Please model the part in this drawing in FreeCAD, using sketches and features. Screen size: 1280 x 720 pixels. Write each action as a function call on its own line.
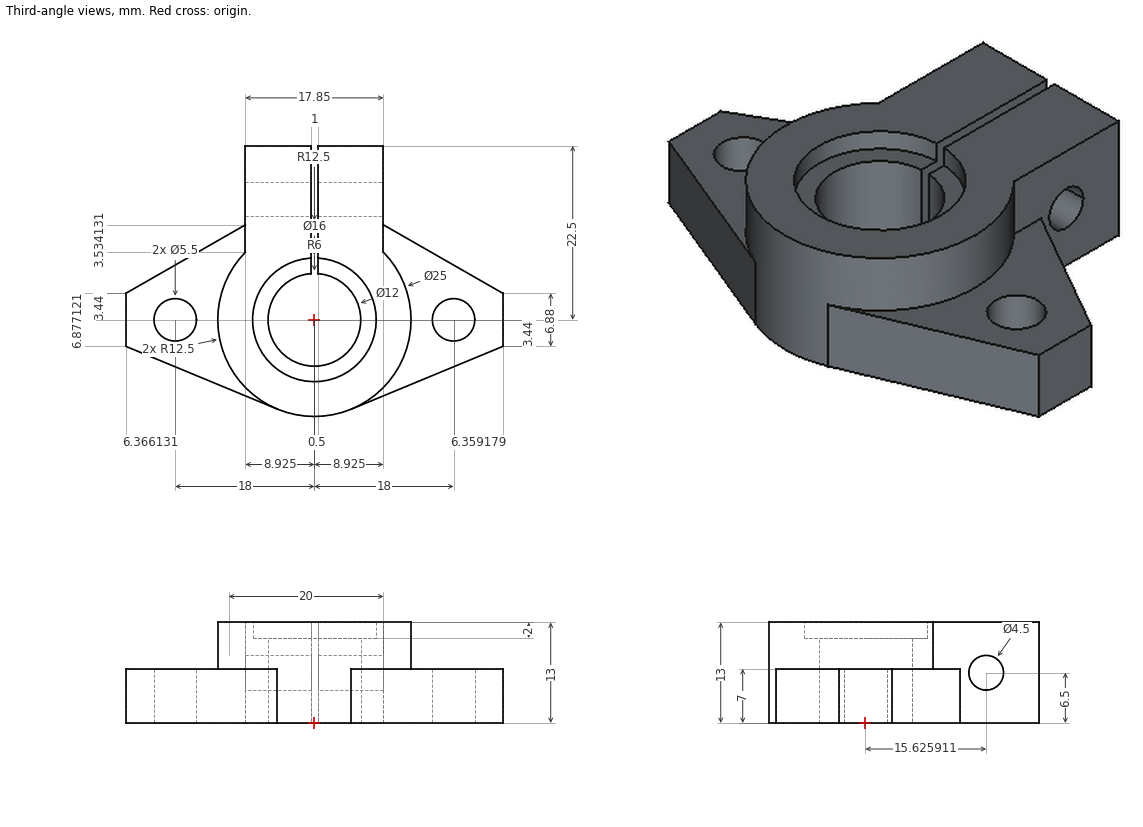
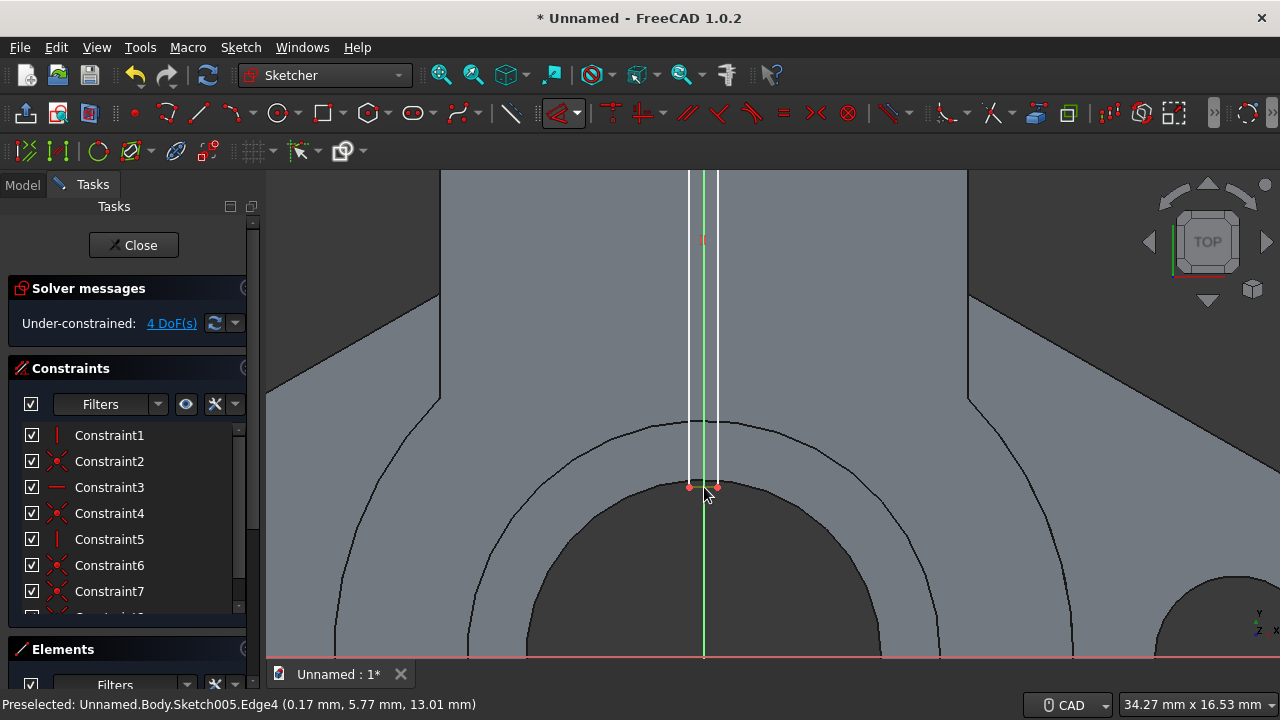
click(580, 114)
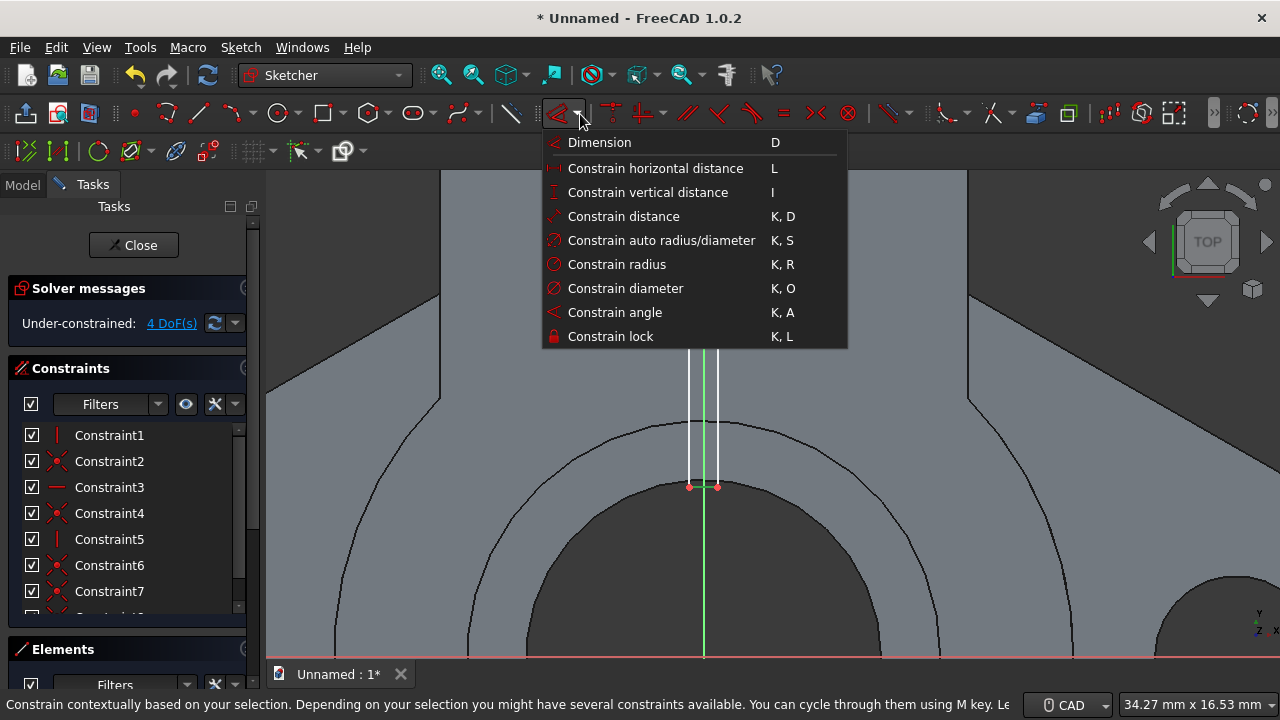
click(695, 264)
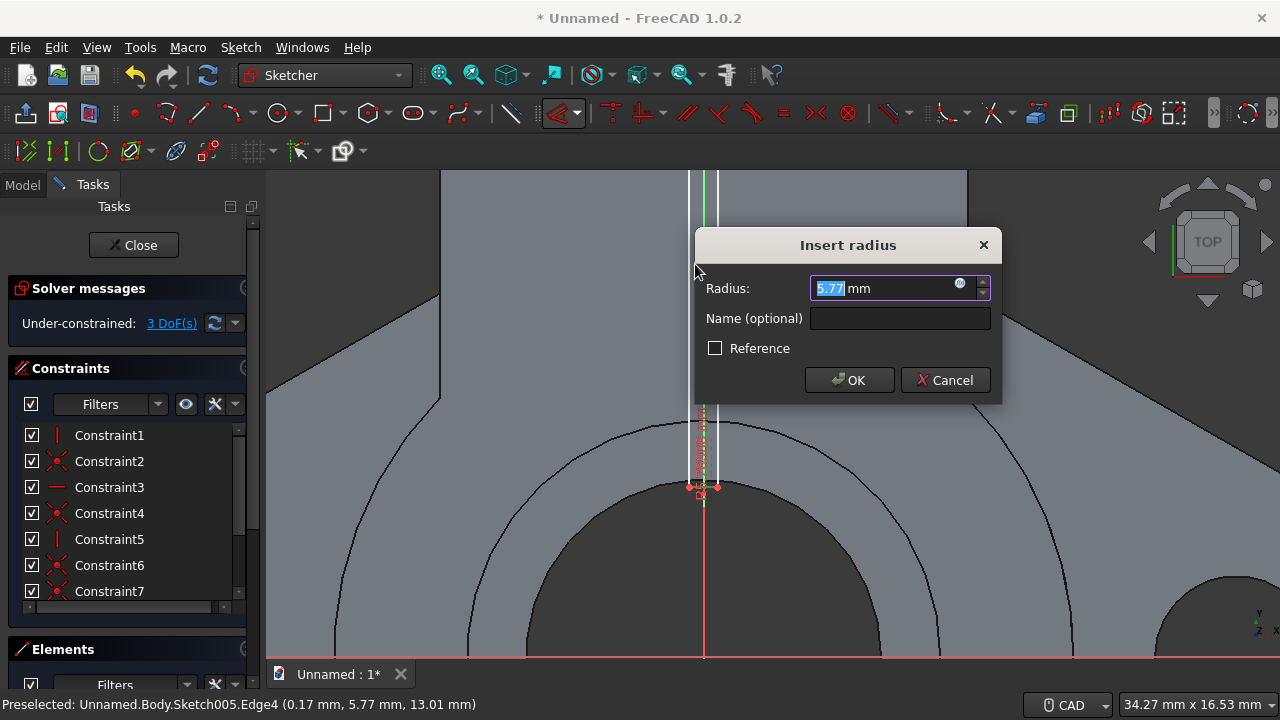
text(6)
key(Return)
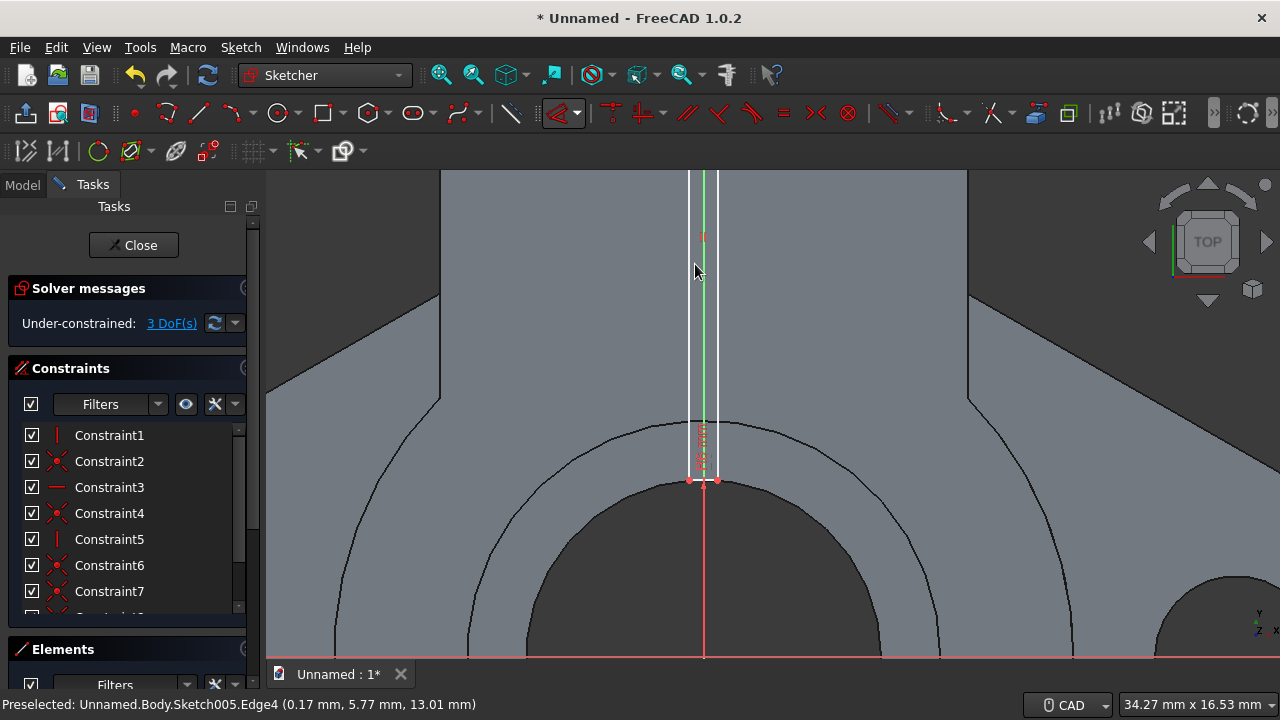
scroll(705, 488, down, 4)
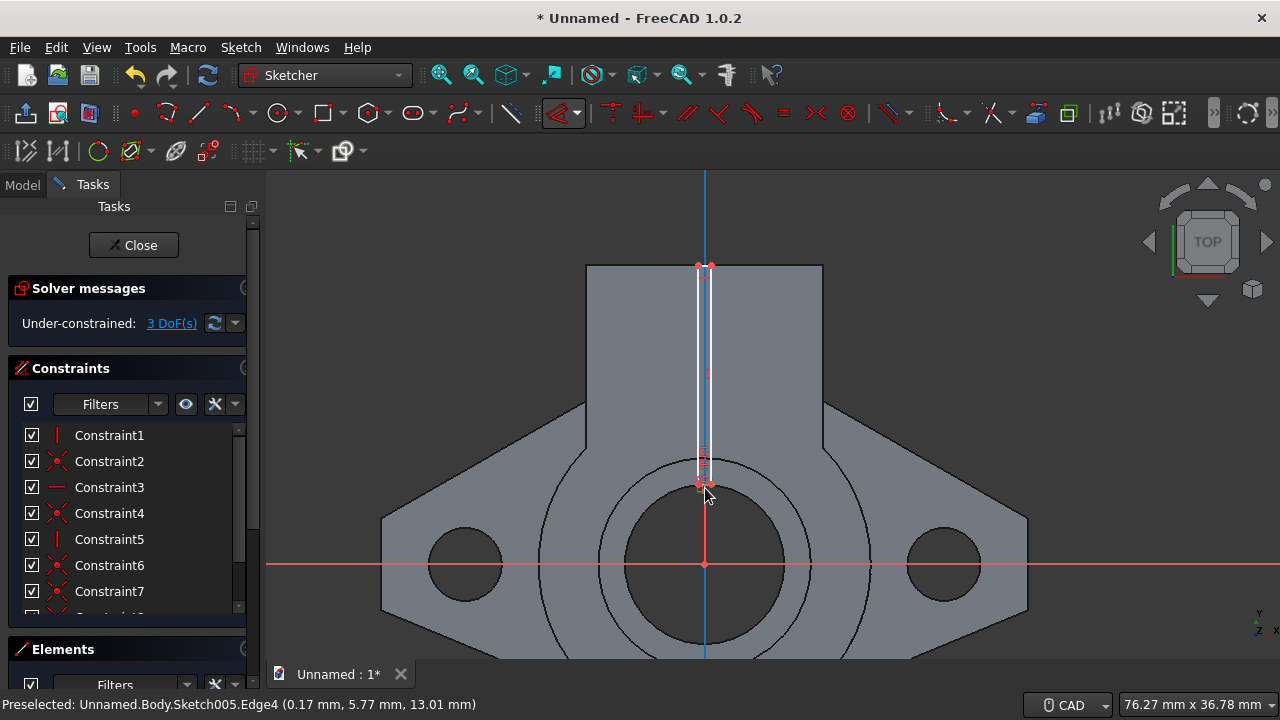
scroll(706, 266, up, 6)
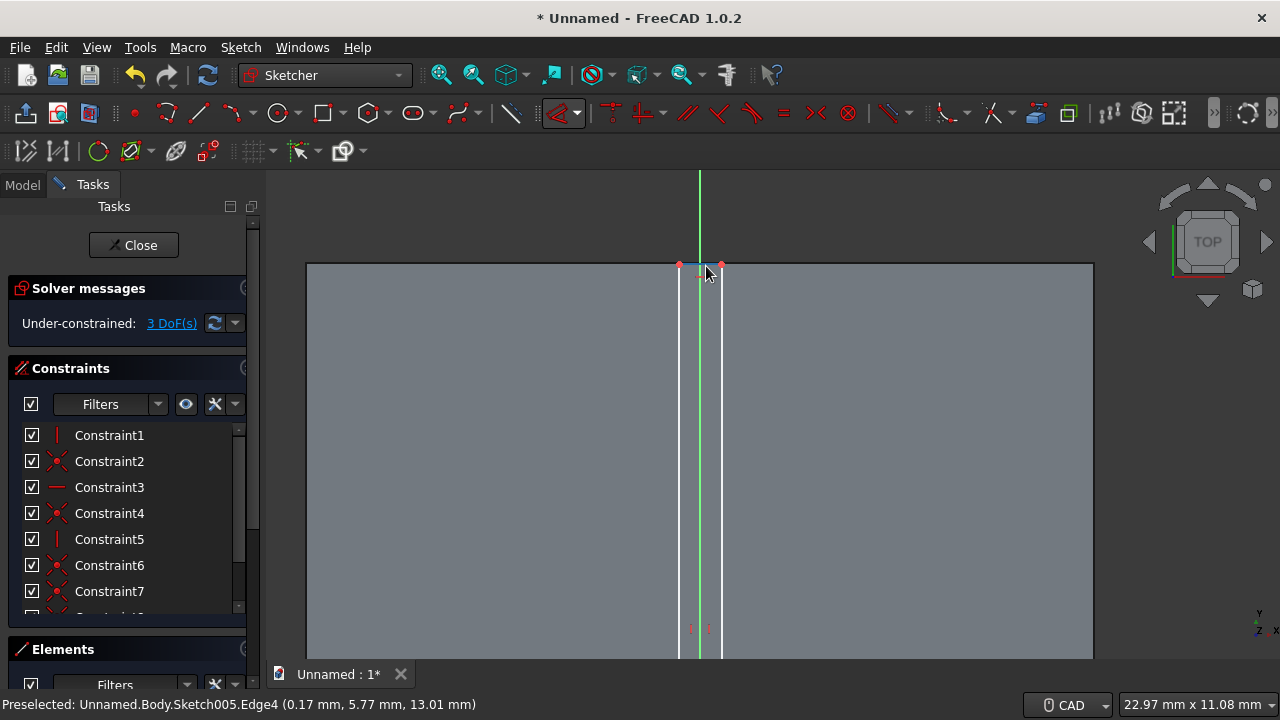
click(705, 264)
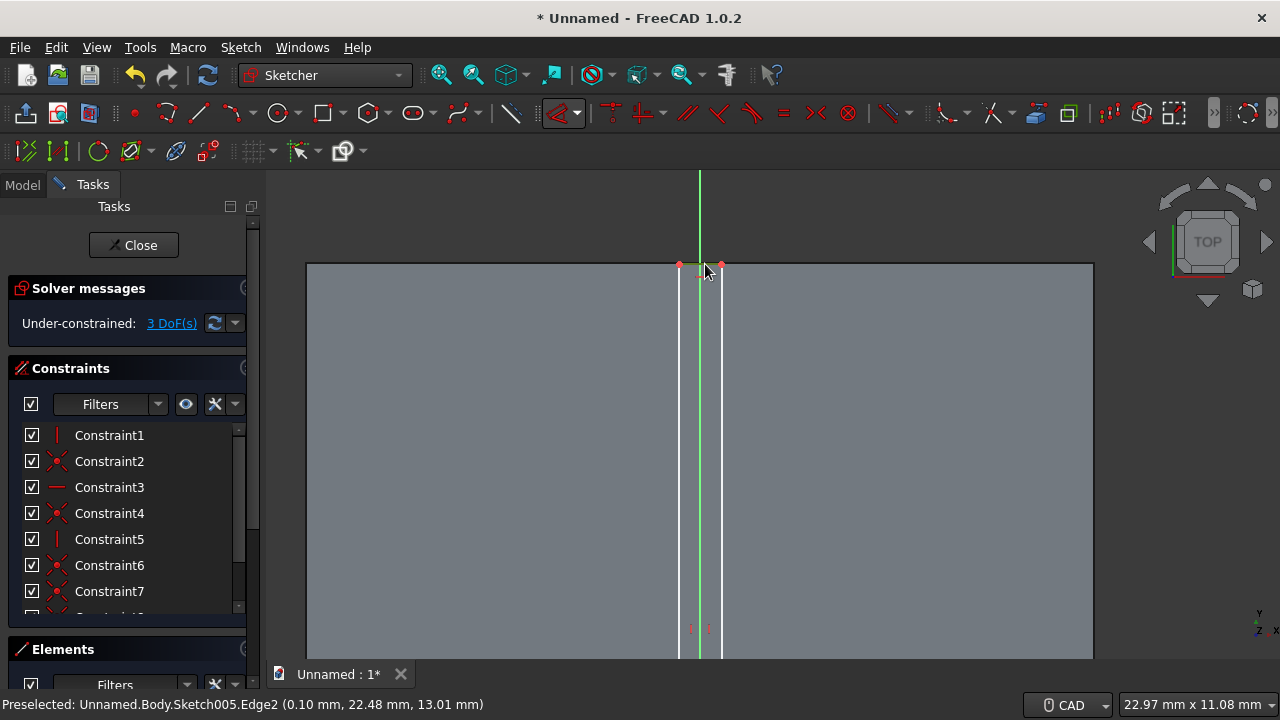
key(l)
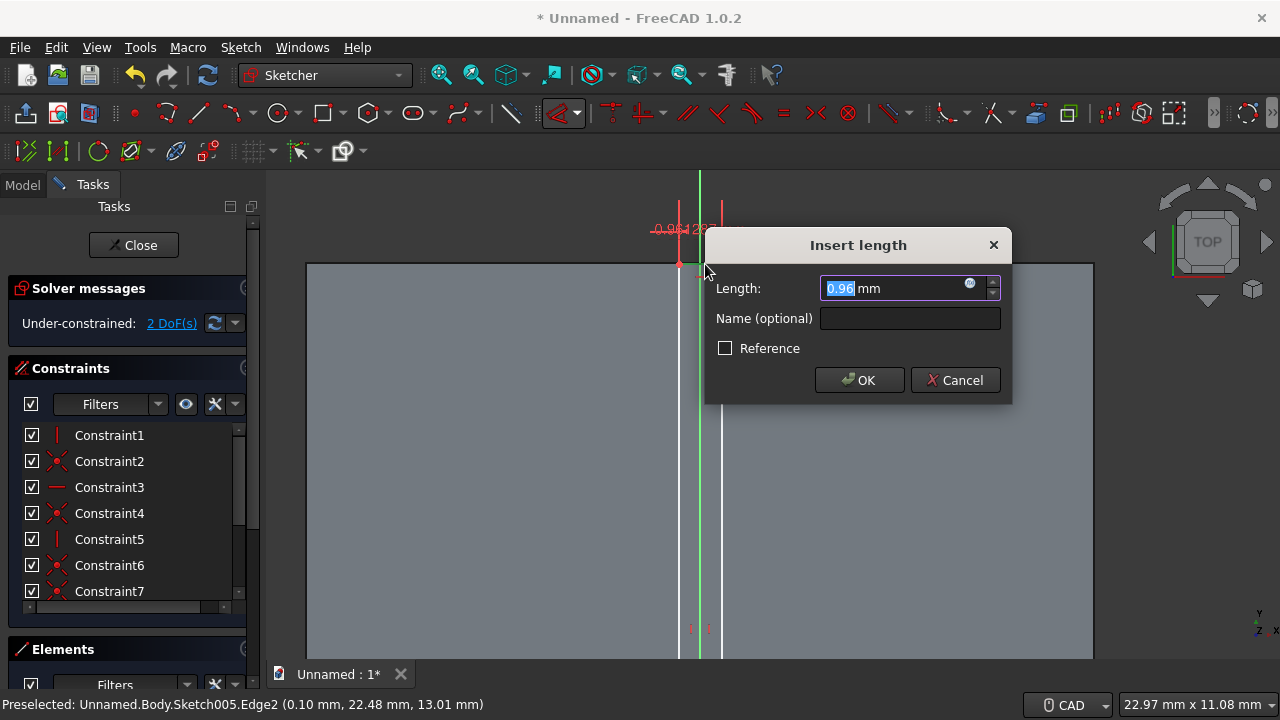
text(1)
key(Return)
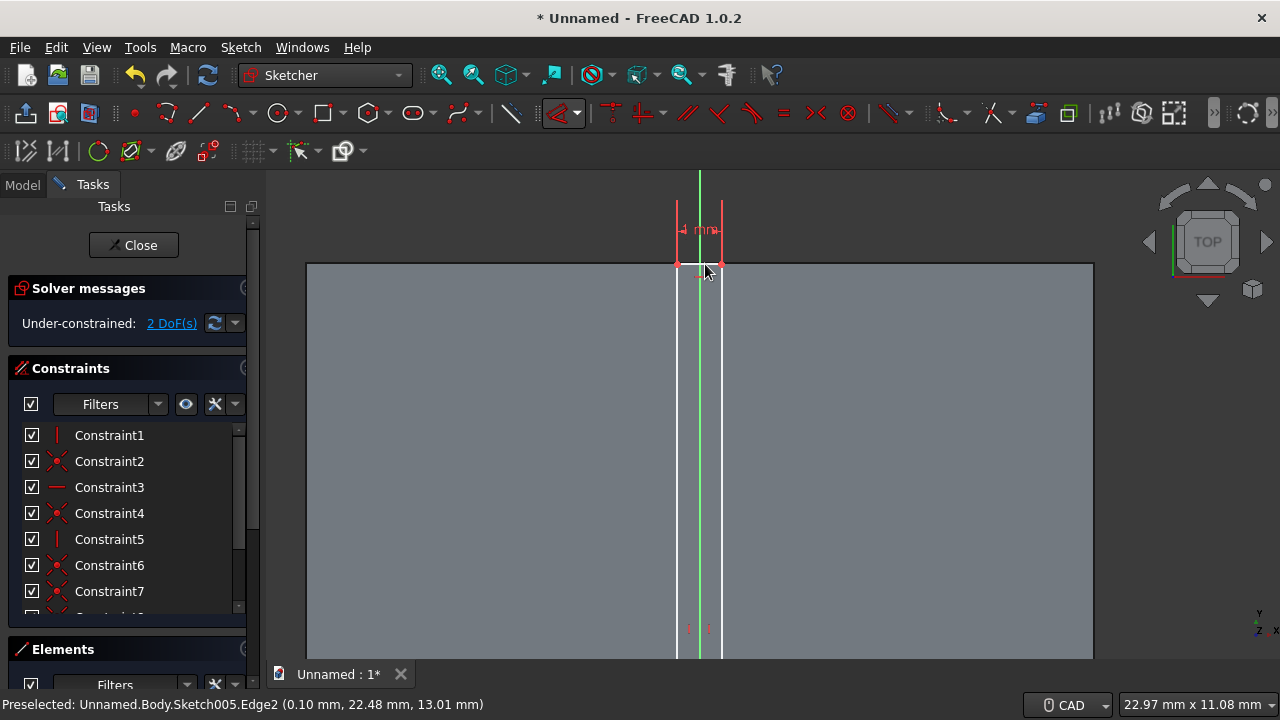
scroll(706, 266, down, 6)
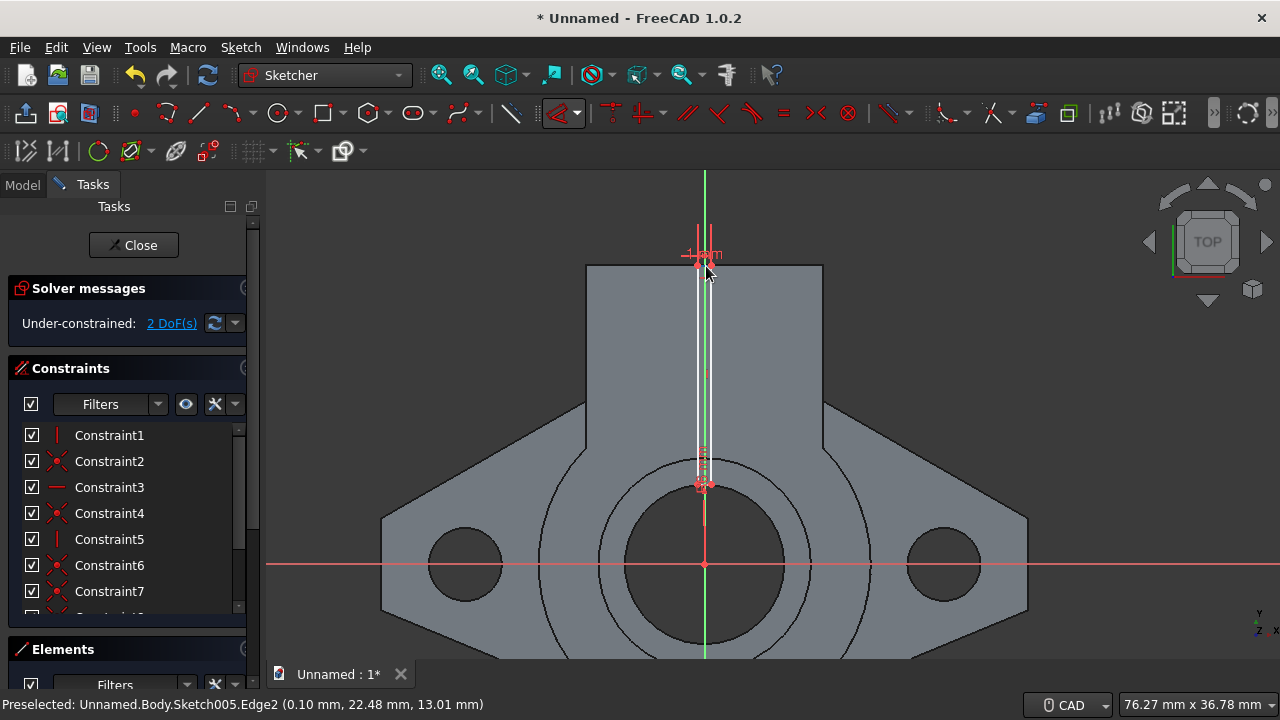
scroll(711, 485, up, 9)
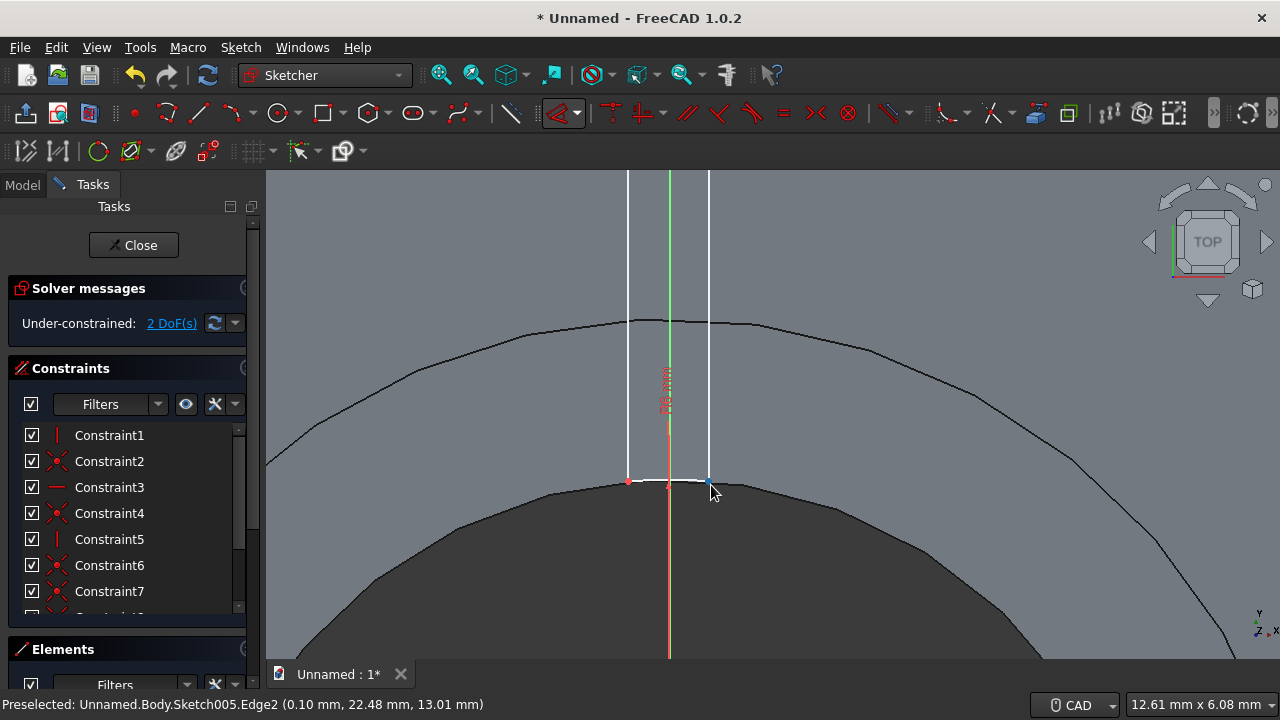
click(709, 481)